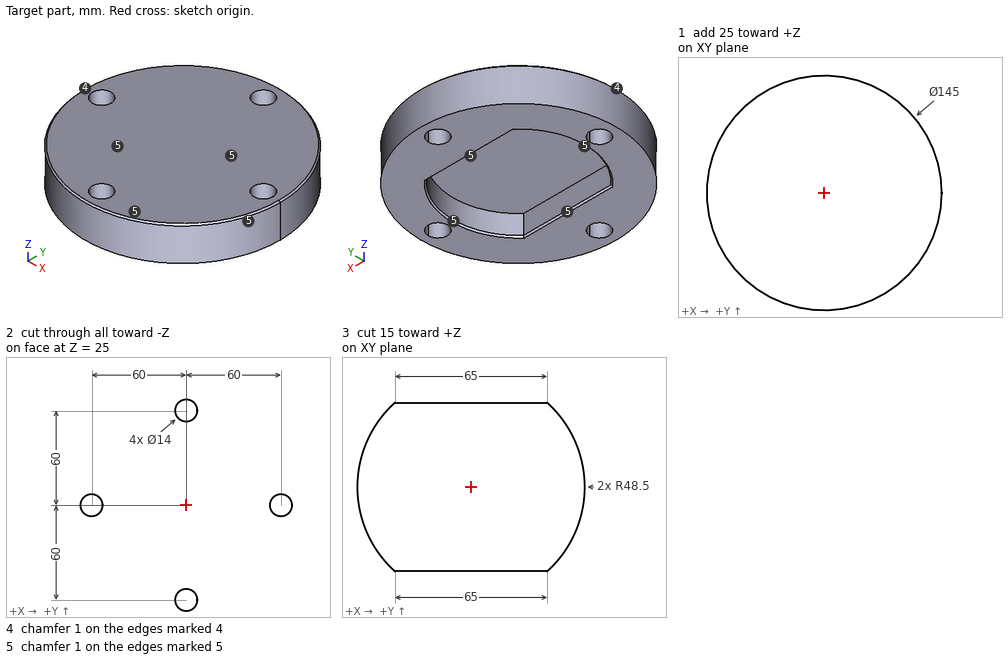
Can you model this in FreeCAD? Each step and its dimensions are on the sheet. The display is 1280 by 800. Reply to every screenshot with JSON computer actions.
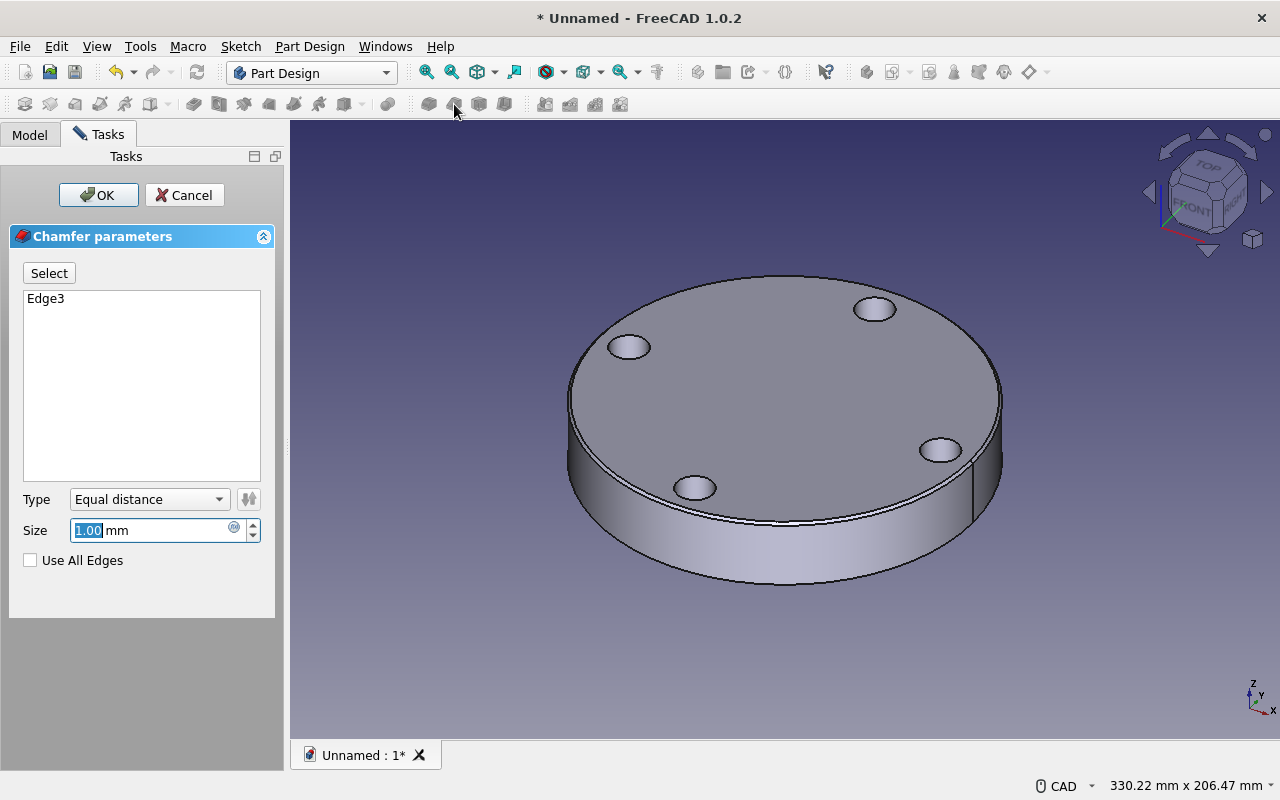
{"action": "type", "text": "1"}
{"action": "key", "text": "Tab"}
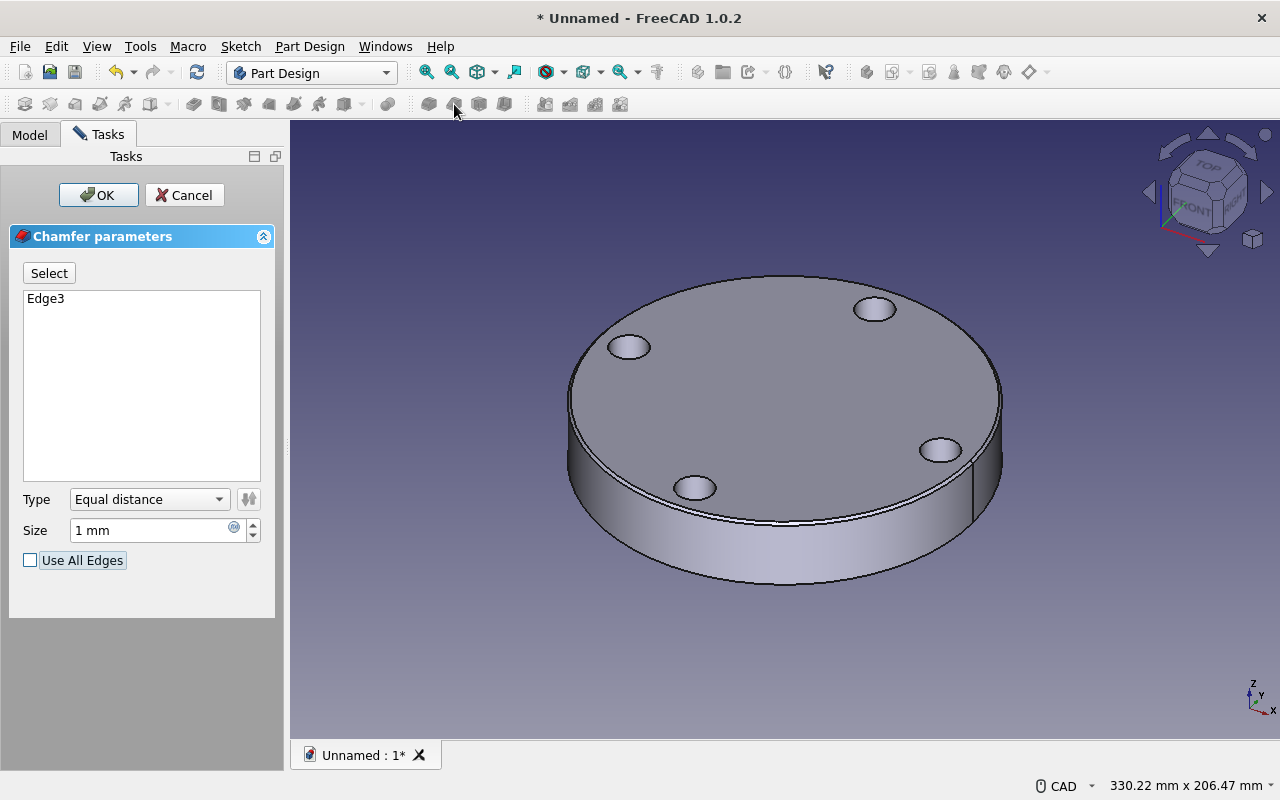
{"action": "left_click", "coordinate": [99, 195]}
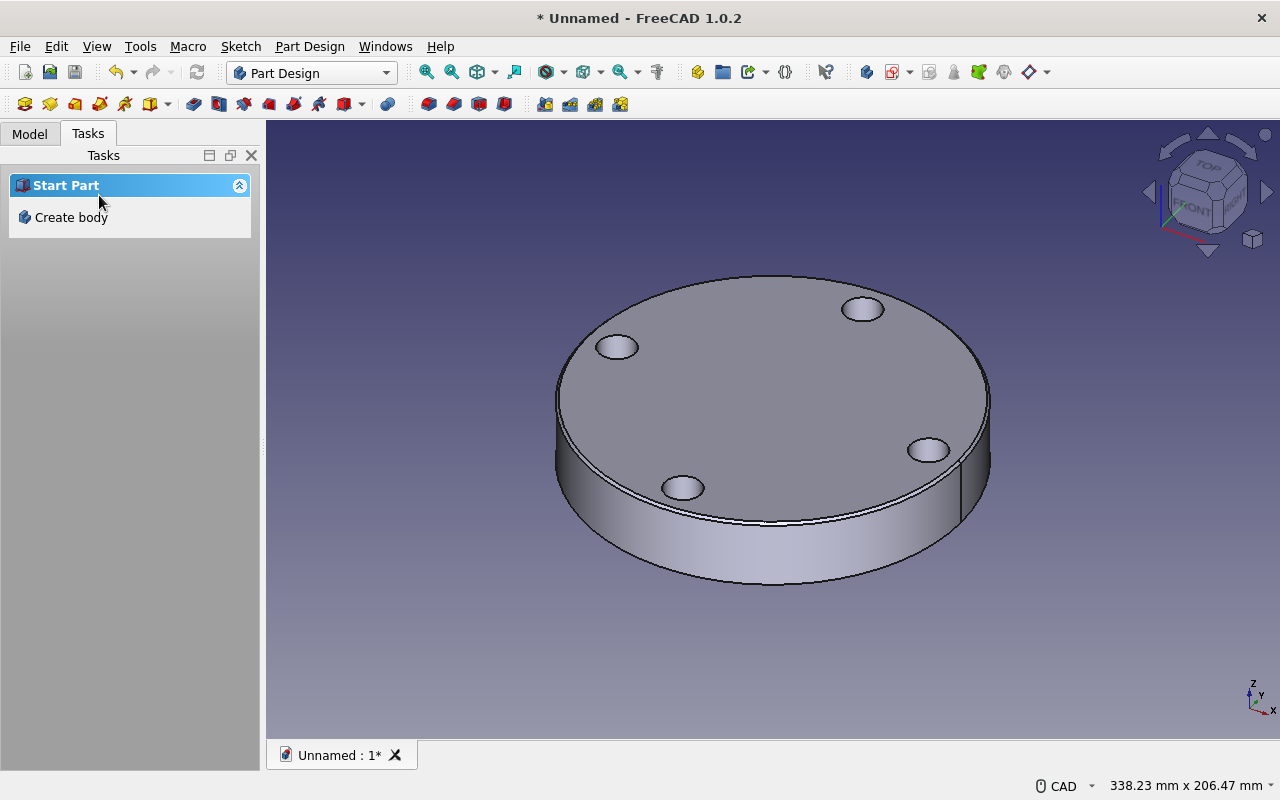
{"action": "key", "text": "0"}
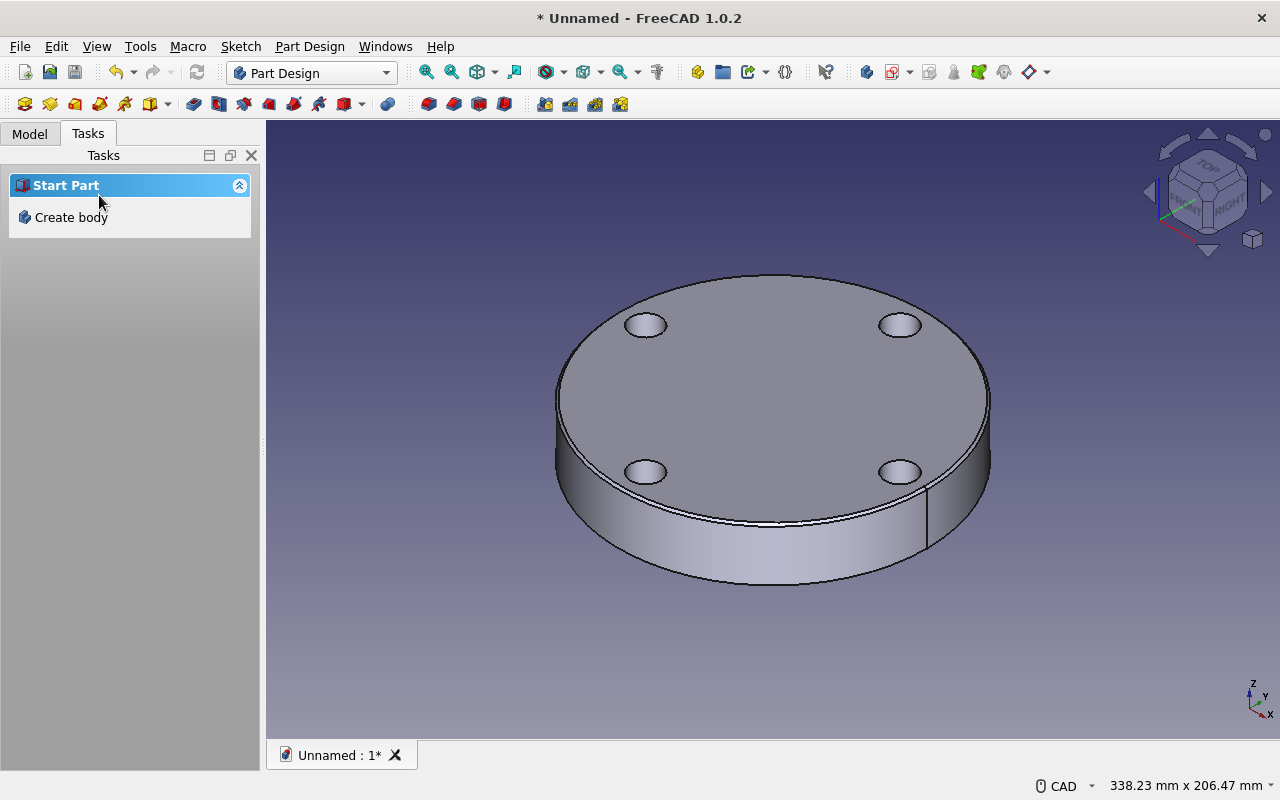
{"action": "key", "text": "2"}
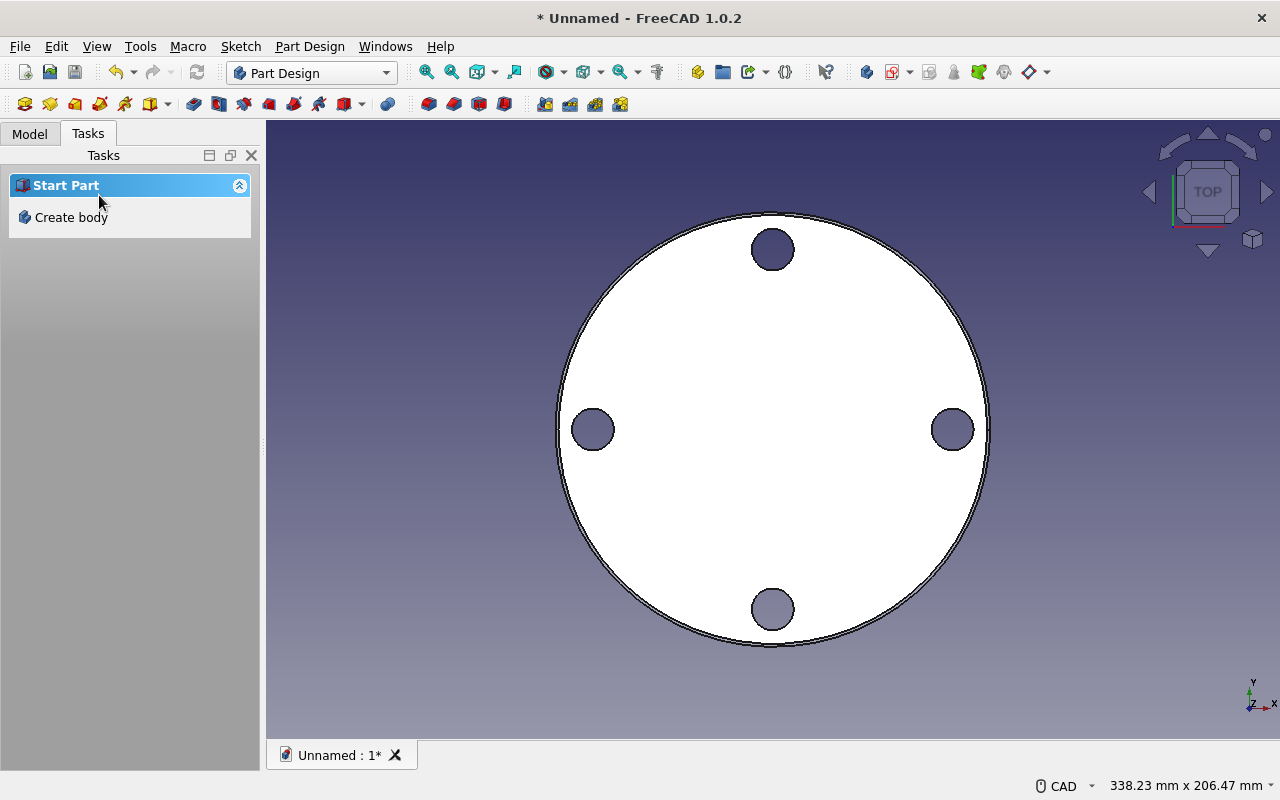
{"action": "key", "text": "1"}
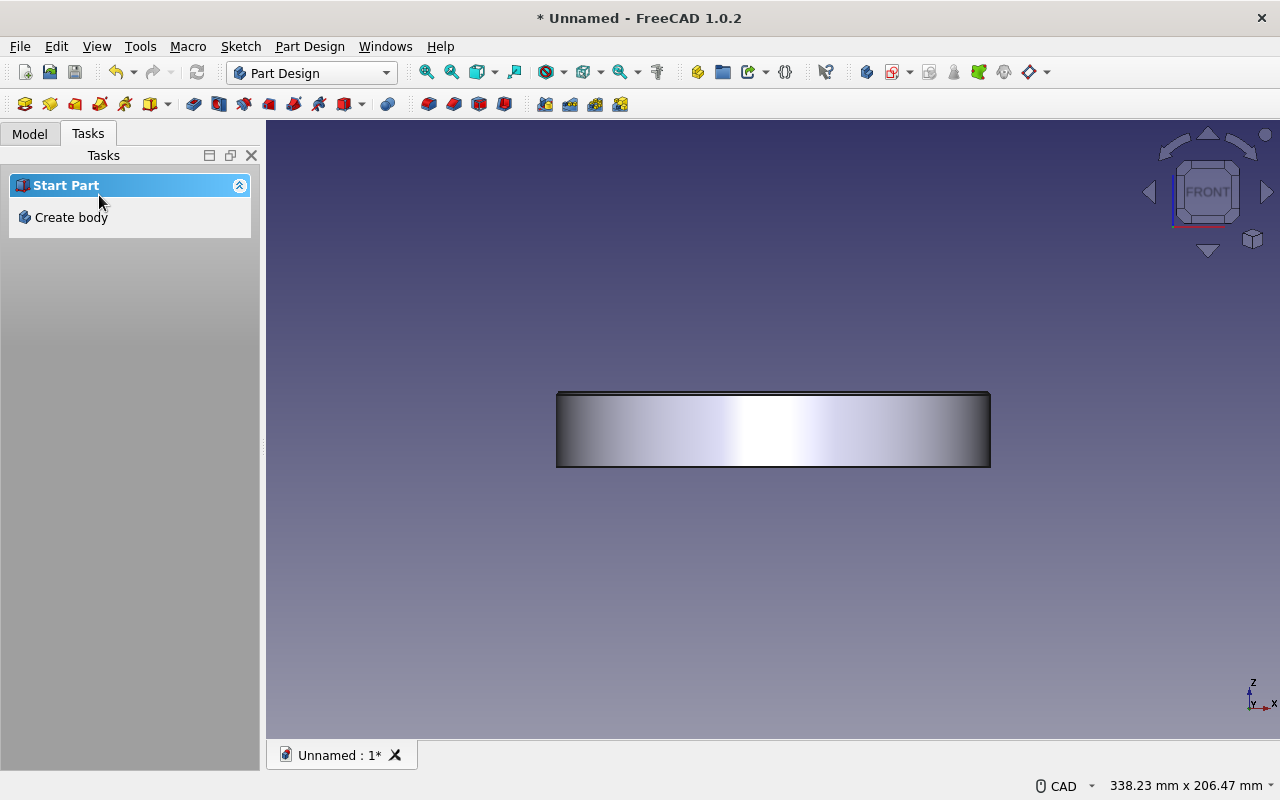
{"action": "left_click", "coordinate": [427, 72]}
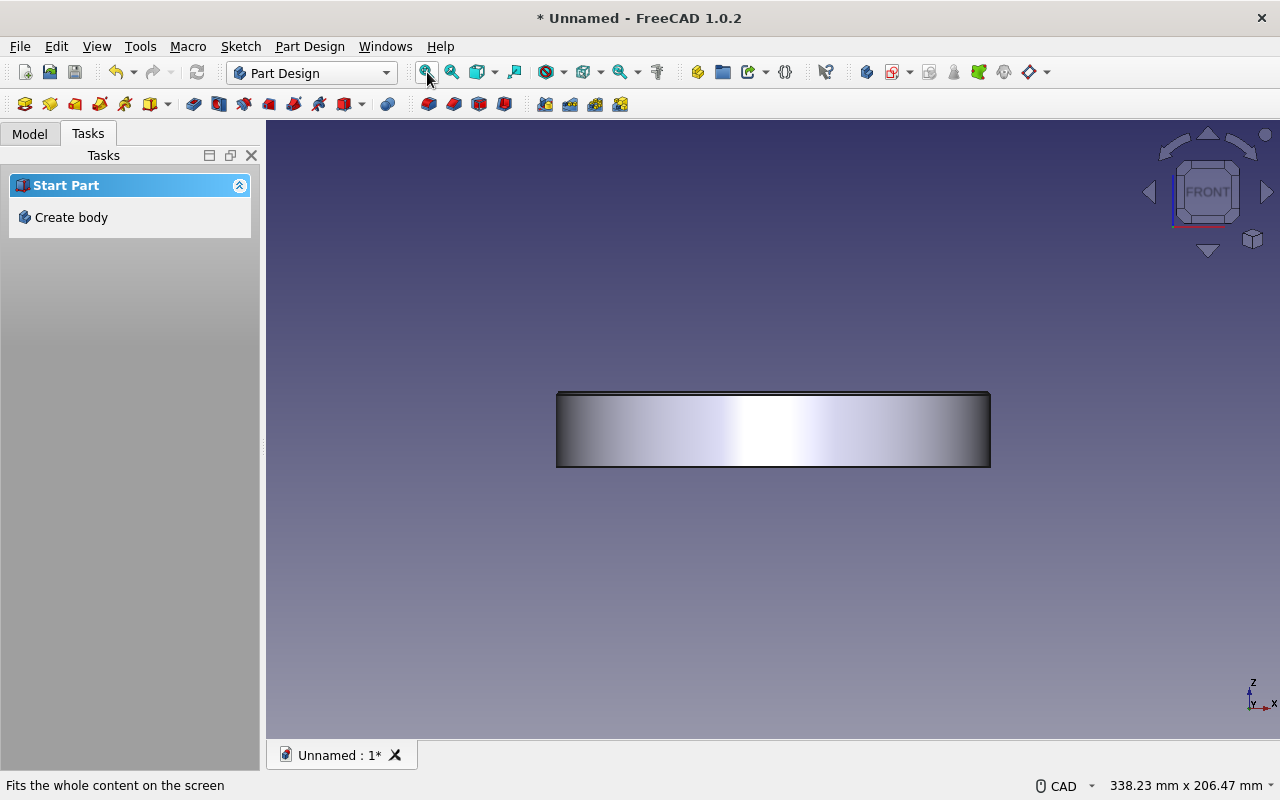
{"action": "key", "text": "3"}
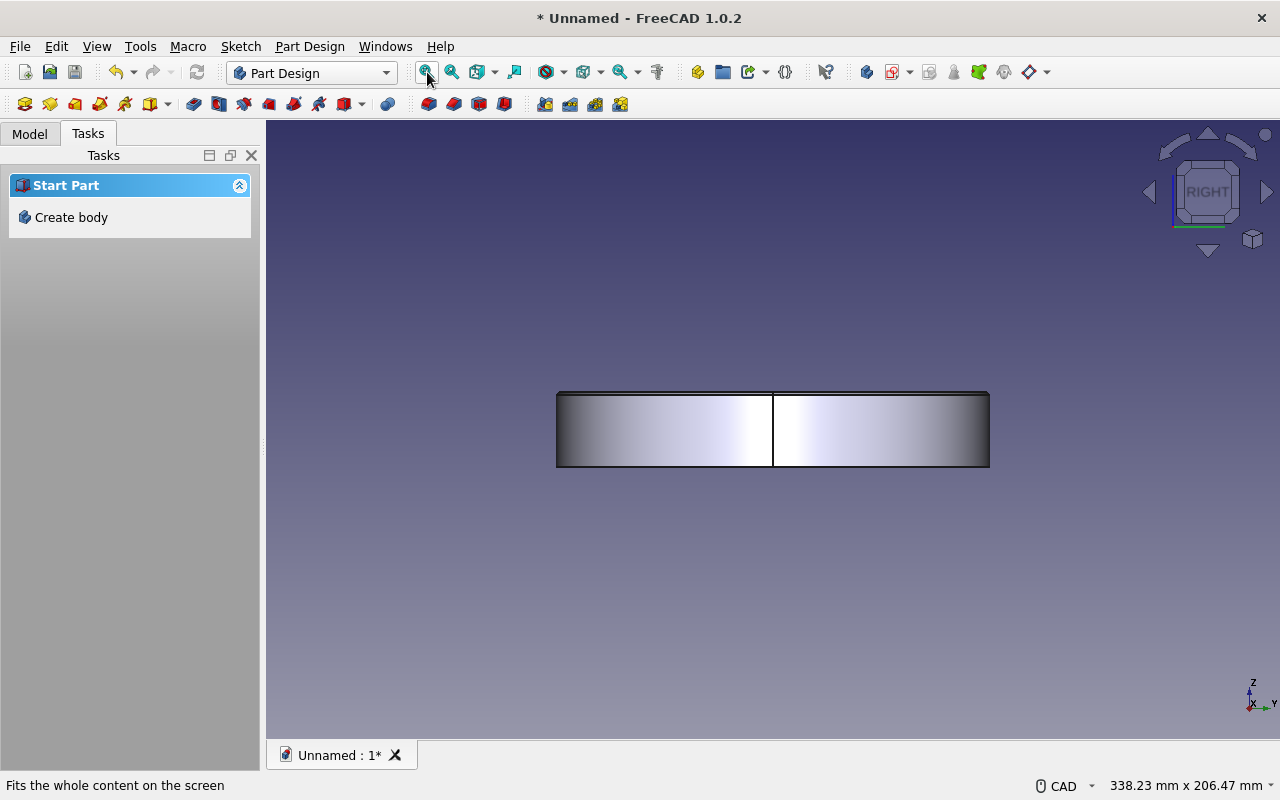
{"action": "left_click", "coordinate": [427, 72]}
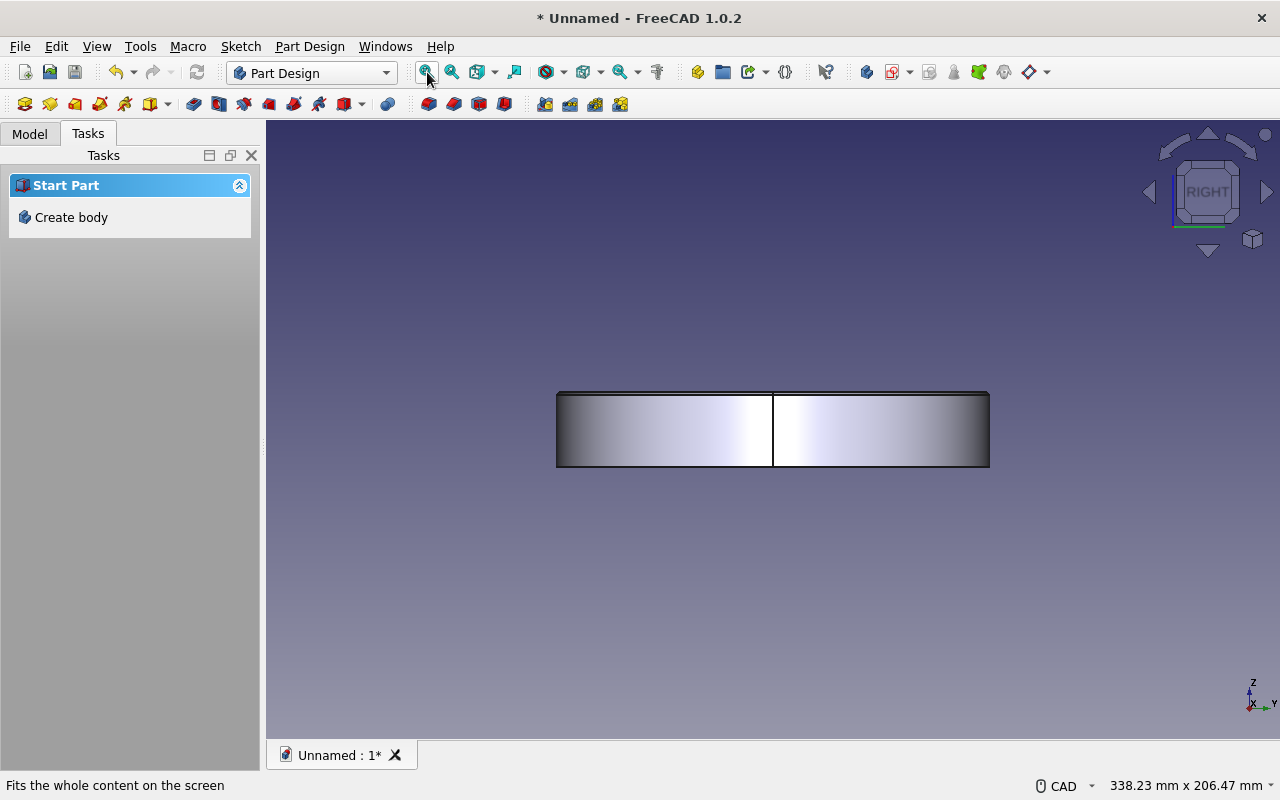
{"action": "key", "text": "5"}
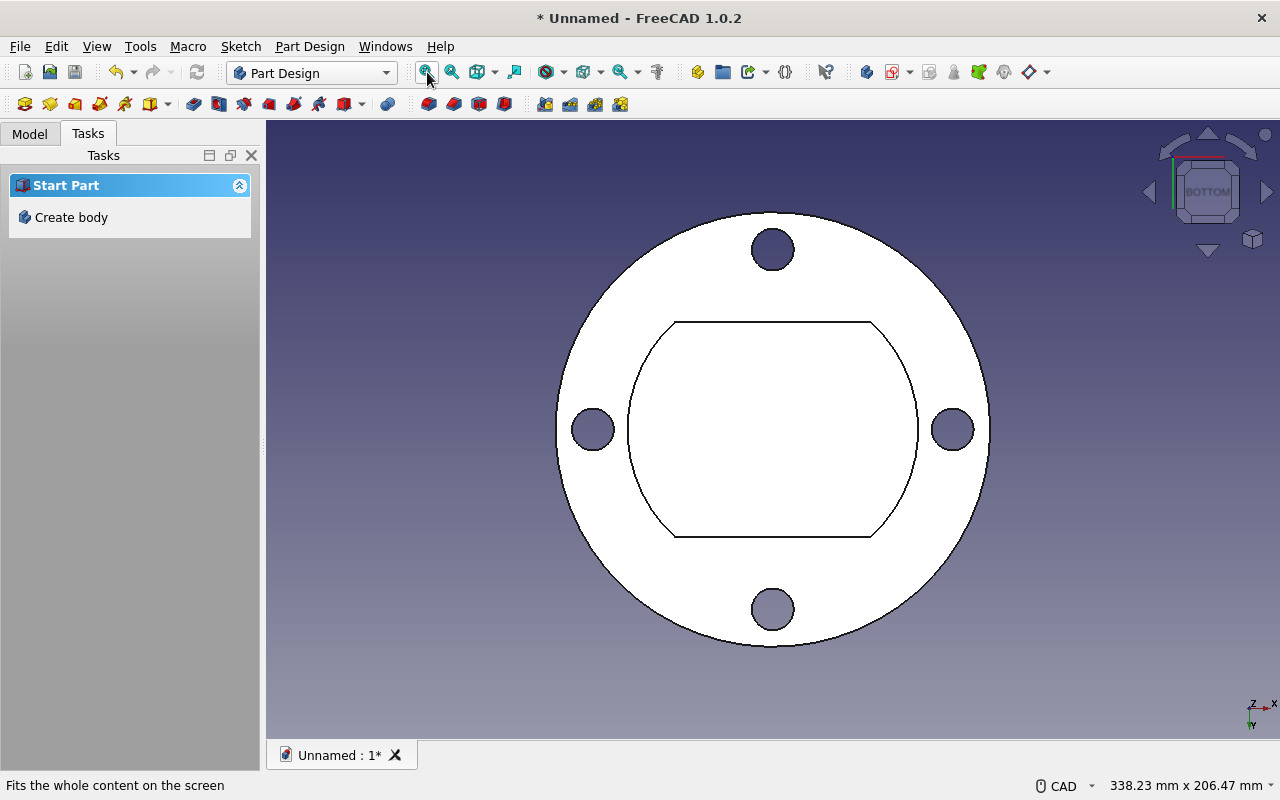
{"action": "left_click", "coordinate": [916, 404]}